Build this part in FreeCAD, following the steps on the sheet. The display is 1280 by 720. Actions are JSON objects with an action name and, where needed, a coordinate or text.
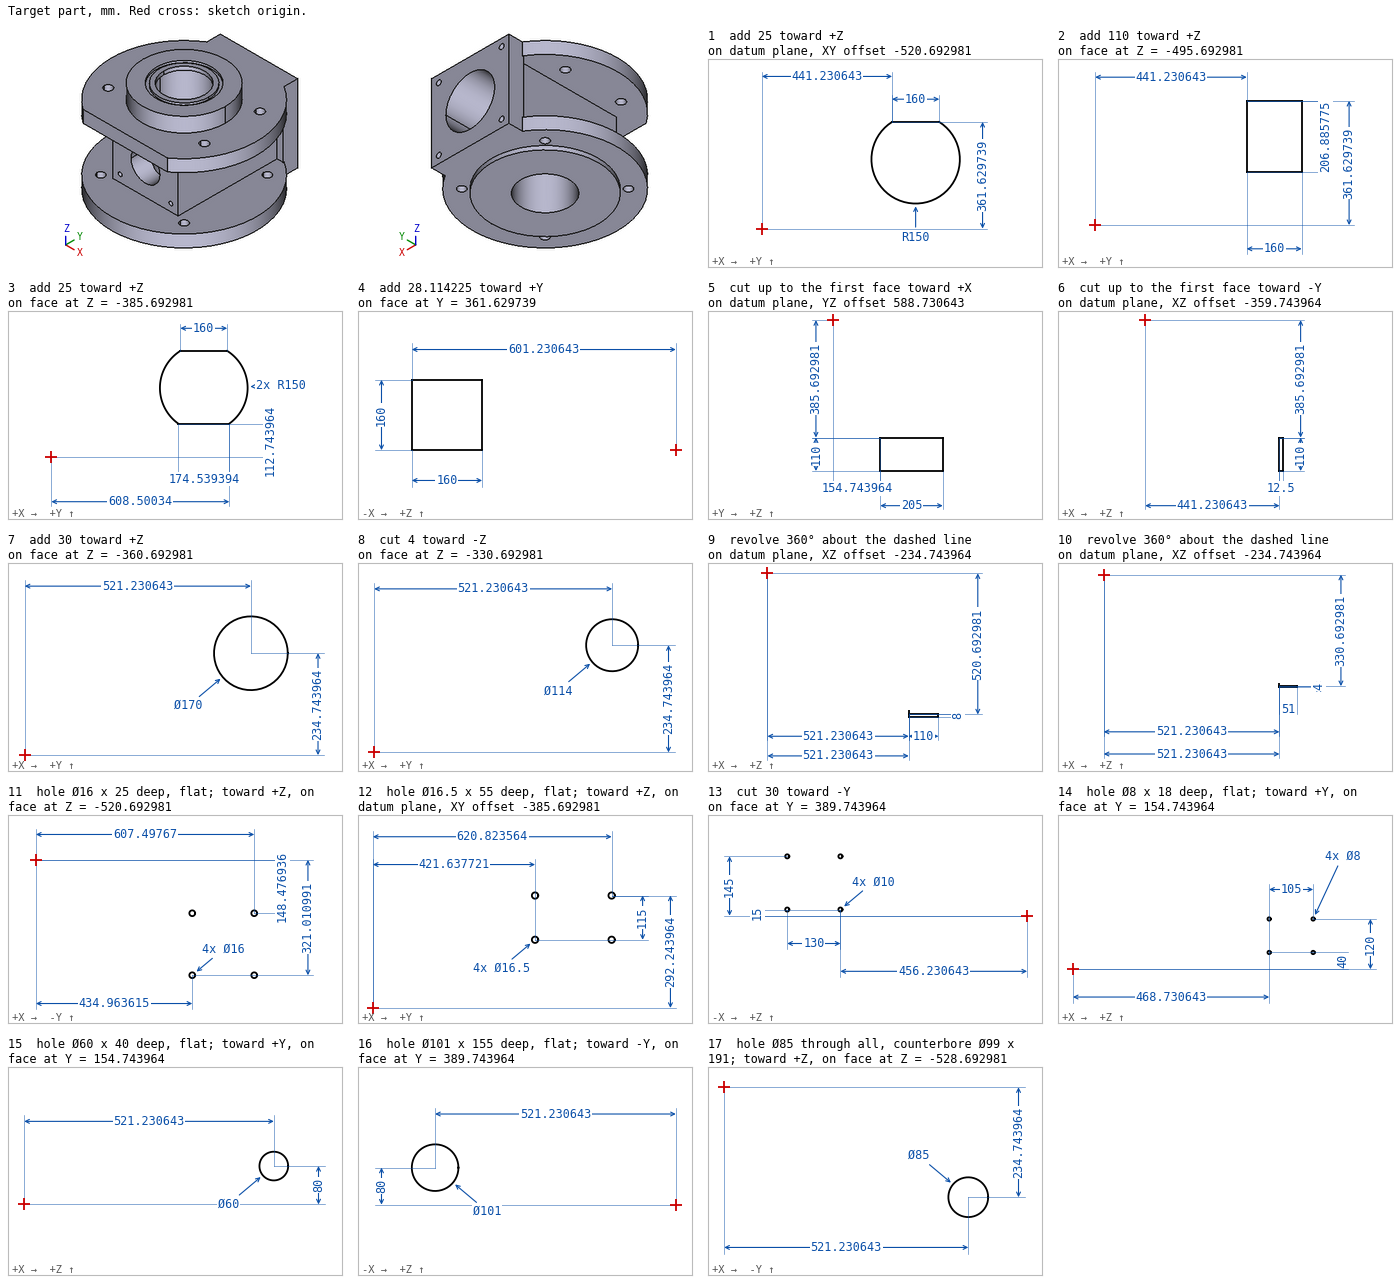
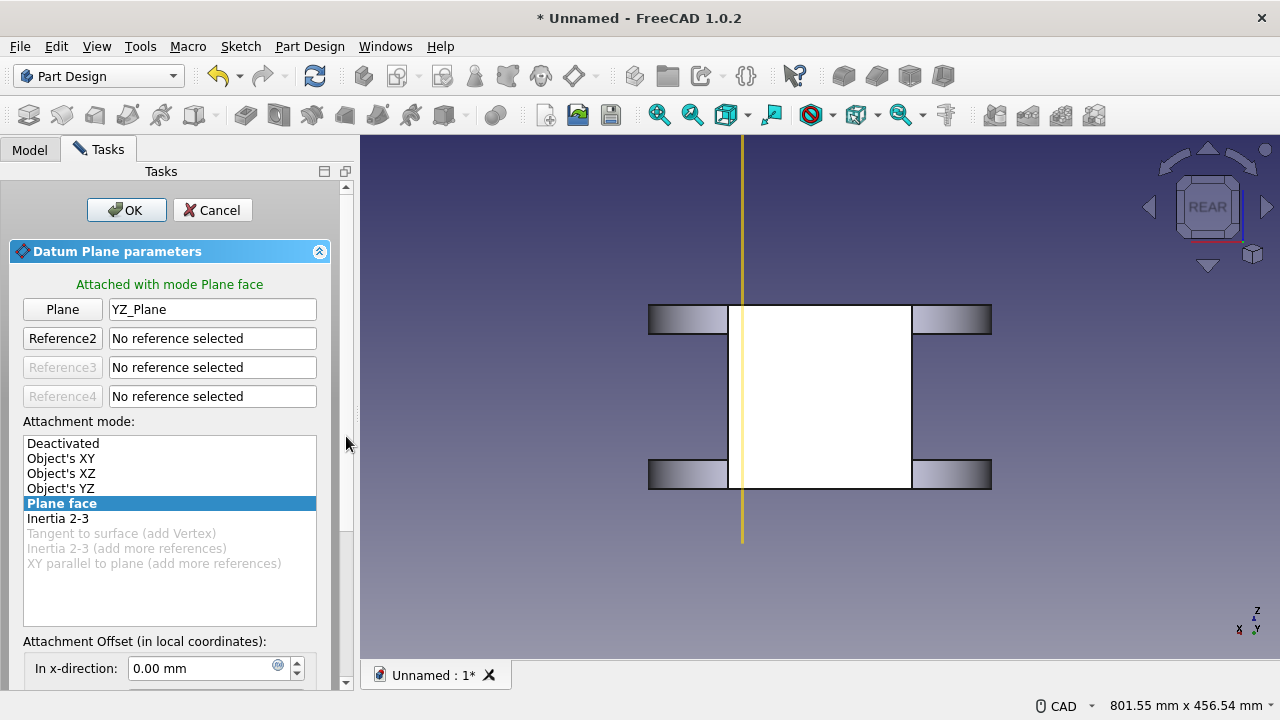
{"action": "left_click", "coordinate": [127, 210]}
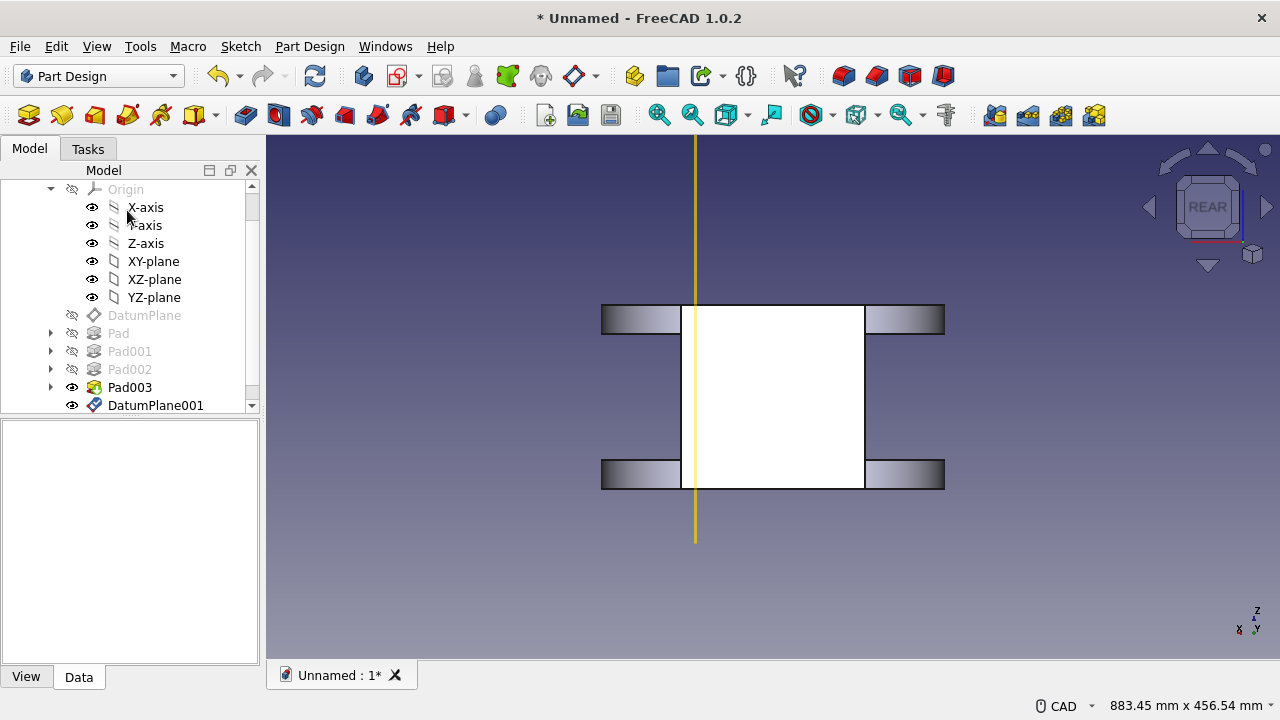
{"action": "left_click", "coordinate": [117, 405]}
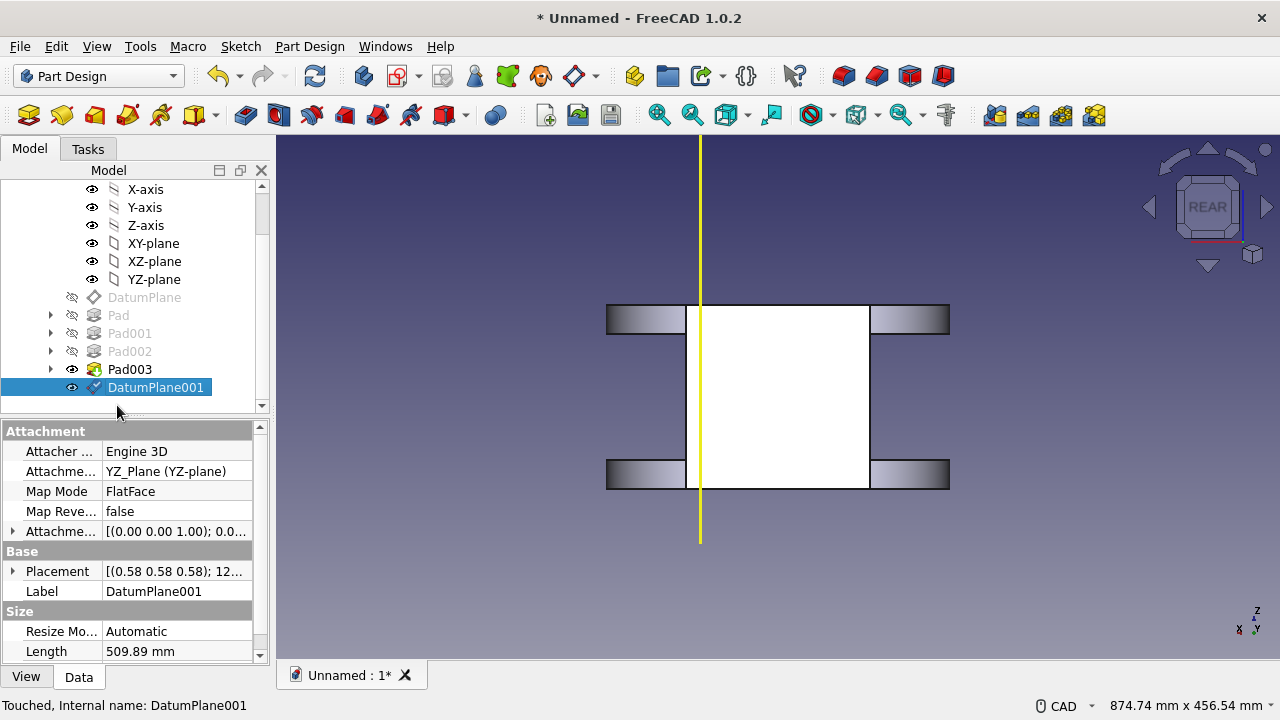
{"action": "left_click", "coordinate": [396, 76]}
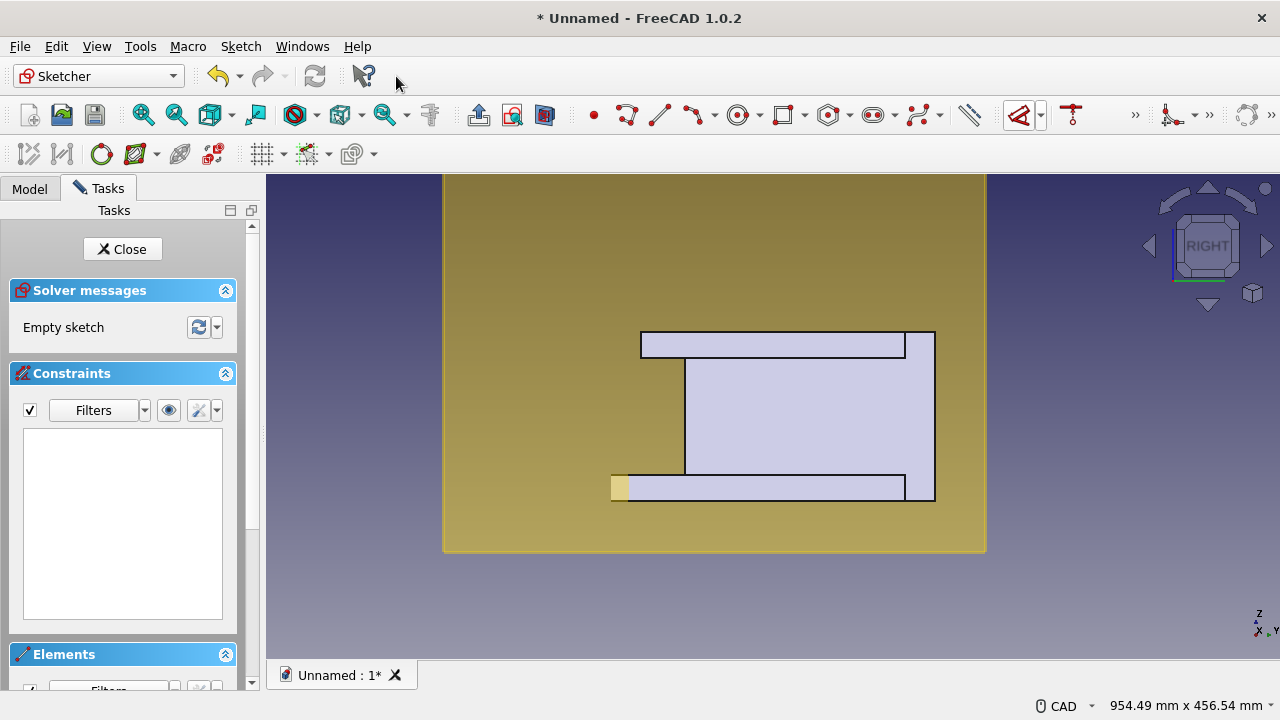
{"action": "left_click", "coordinate": [545, 116]}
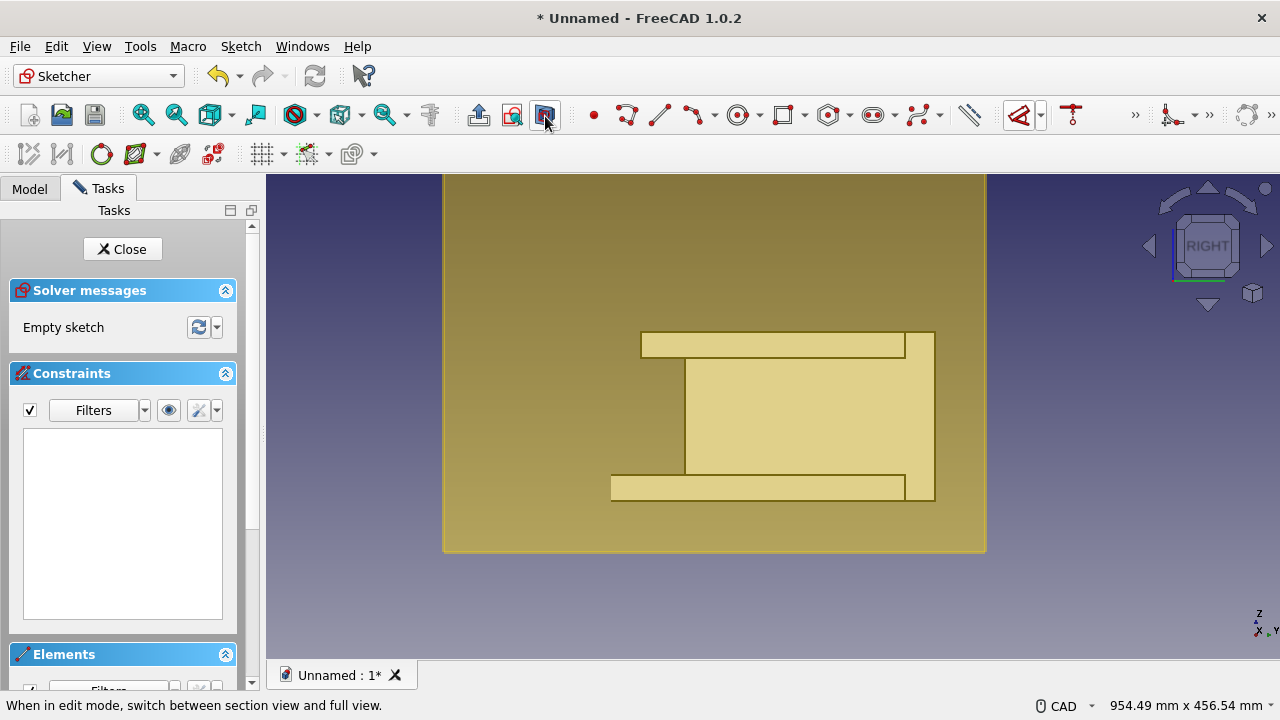
{"action": "scroll", "coordinate": [695, 631], "scroll_direction": "down", "scroll_amount": 3}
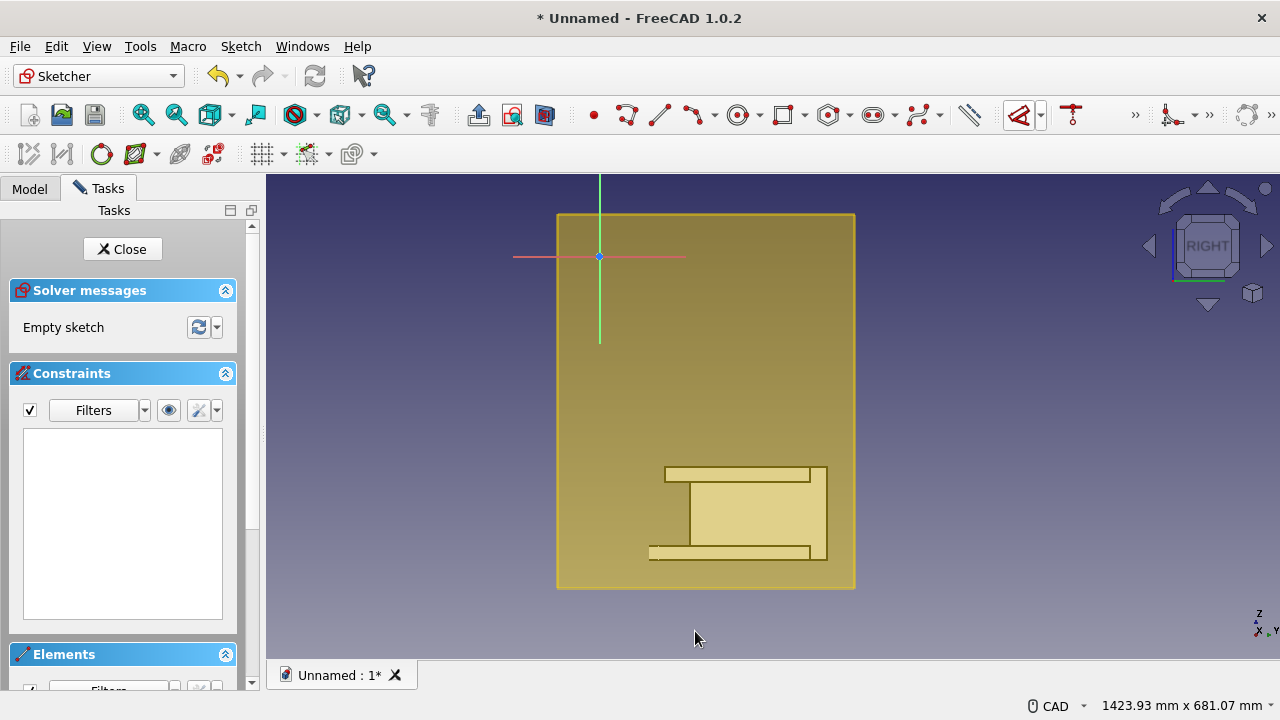
{"action": "left_click", "coordinate": [782, 116]}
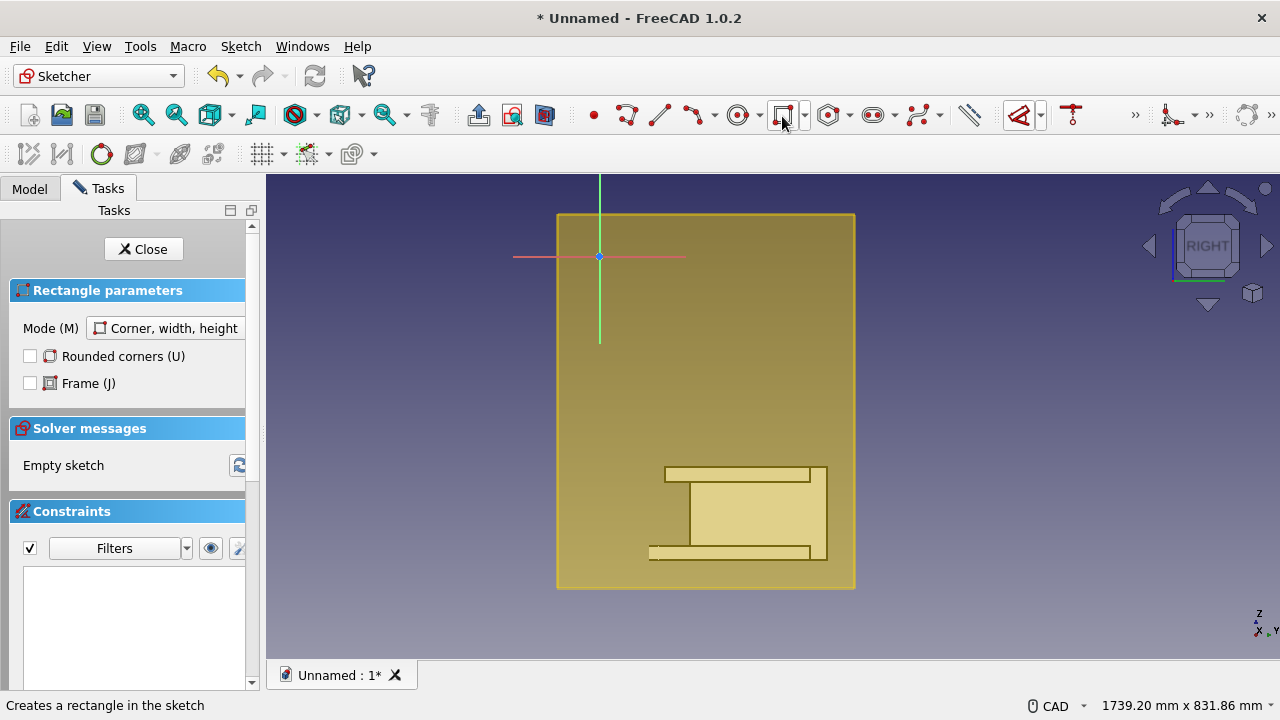
{"action": "left_click", "coordinate": [690, 482]}
{"action": "left_click", "coordinate": [809, 546]}
{"action": "key", "text": "Escape"}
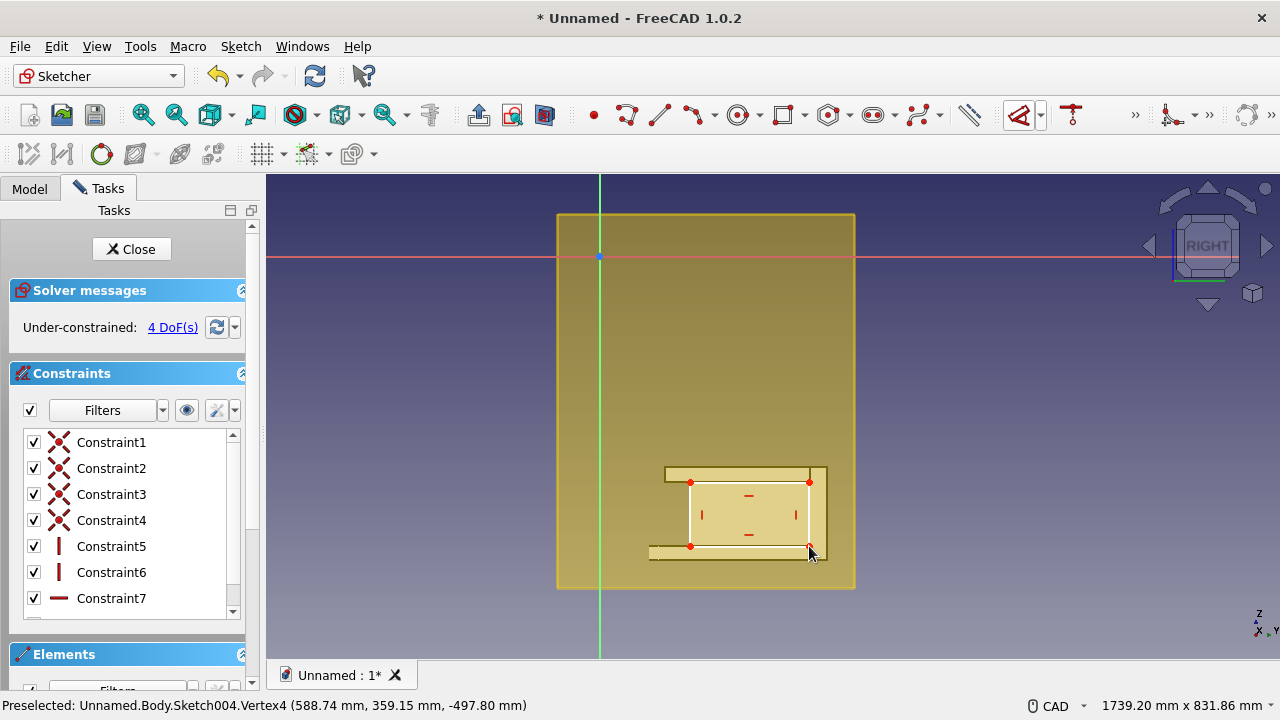
{"action": "left_click", "coordinate": [690, 502]}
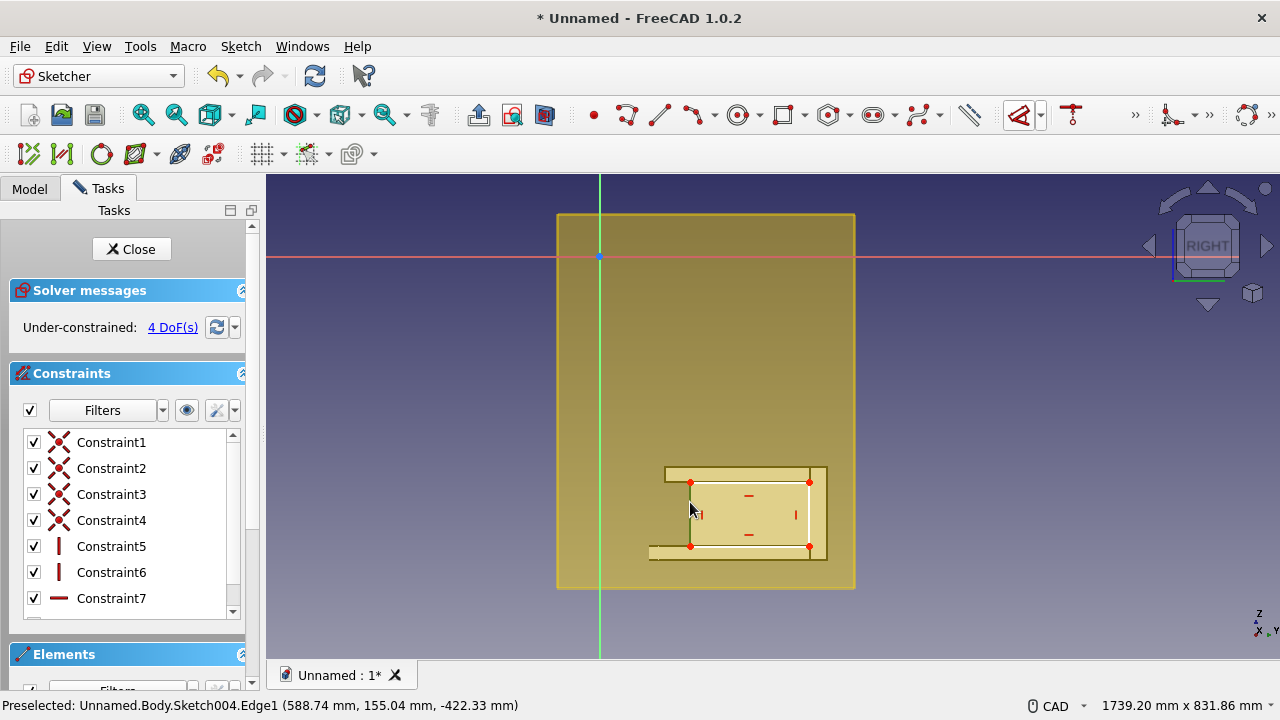
{"action": "left_click", "coordinate": [1040, 116]}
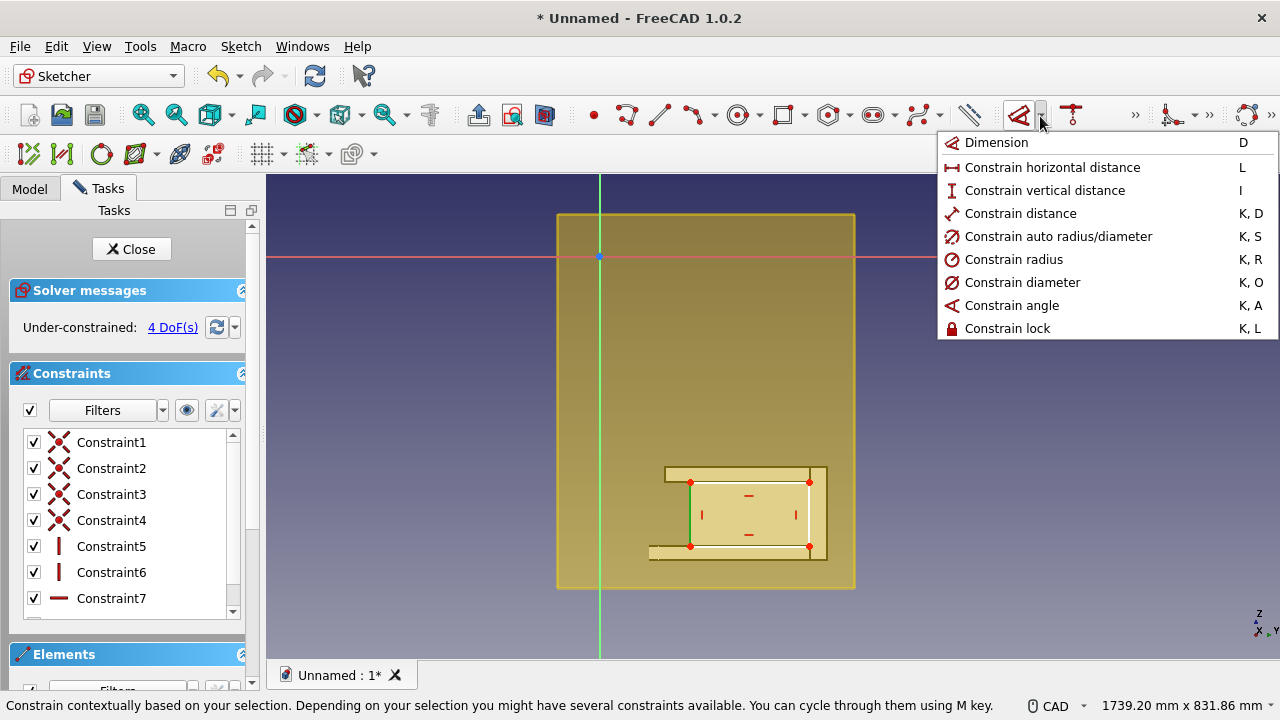
{"action": "left_click", "coordinate": [1108, 190]}